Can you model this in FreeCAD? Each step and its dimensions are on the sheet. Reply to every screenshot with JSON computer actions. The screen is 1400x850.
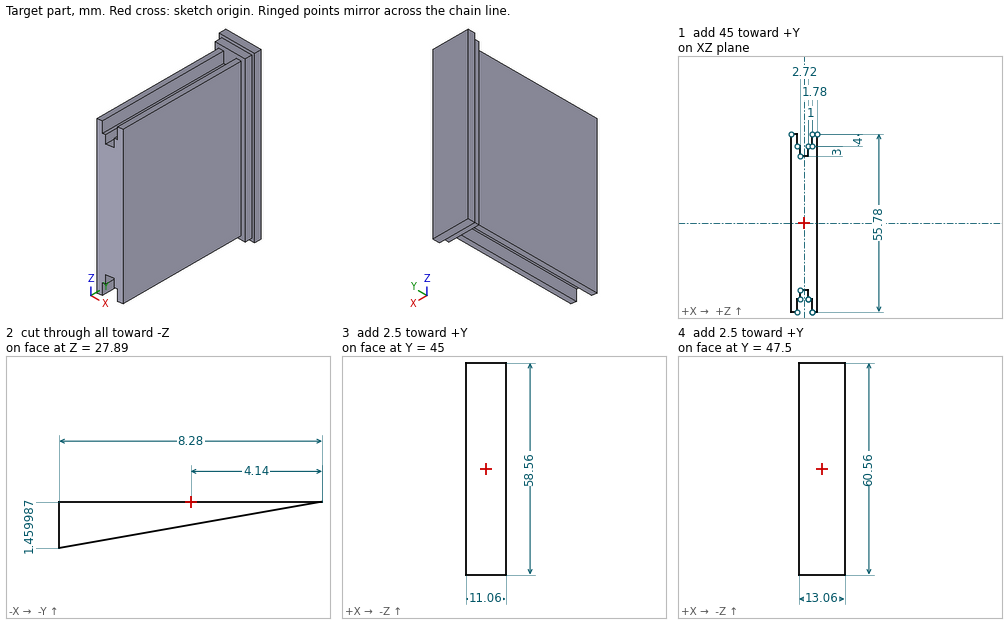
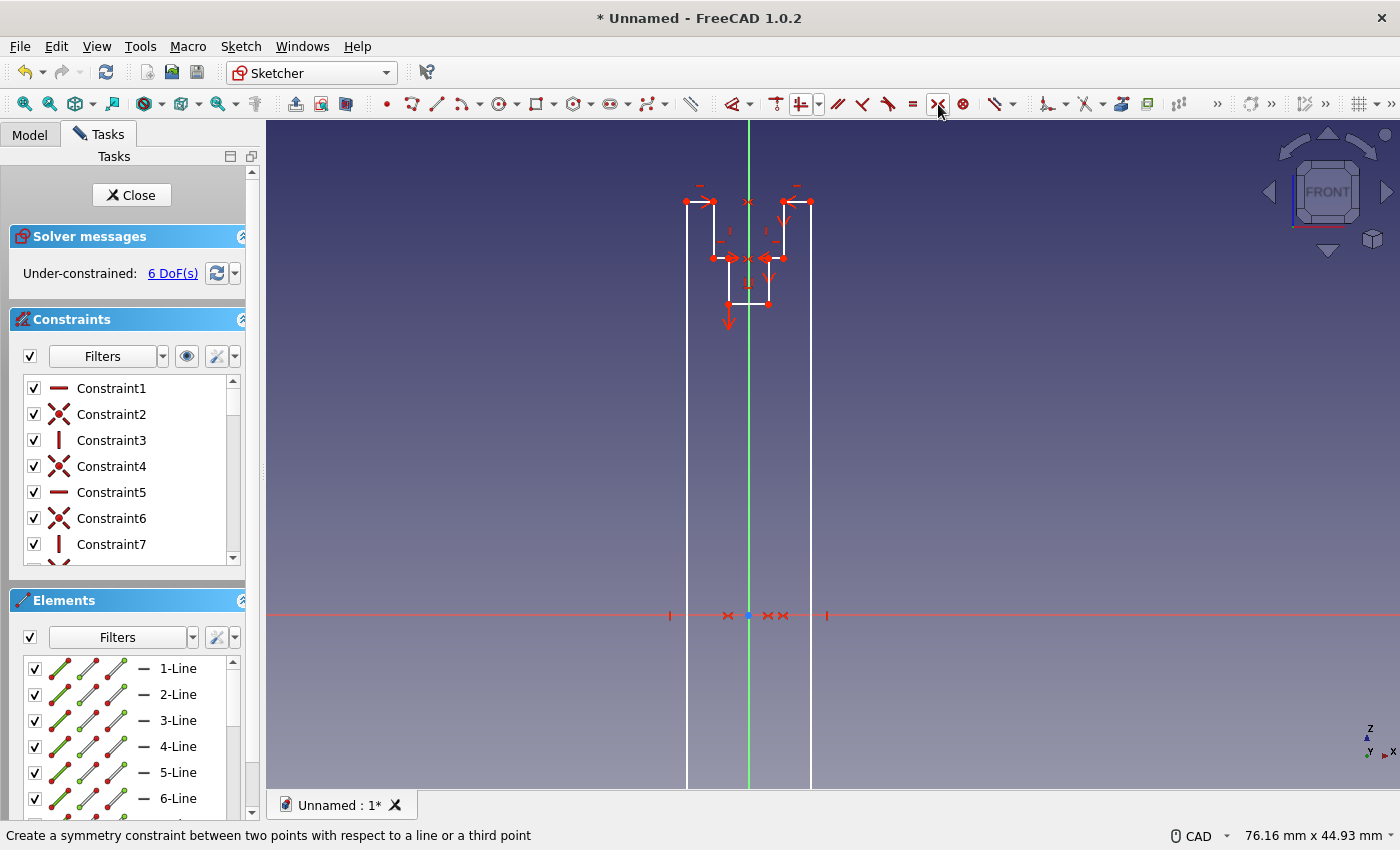
{"action": "left_click", "coordinate": [732, 104]}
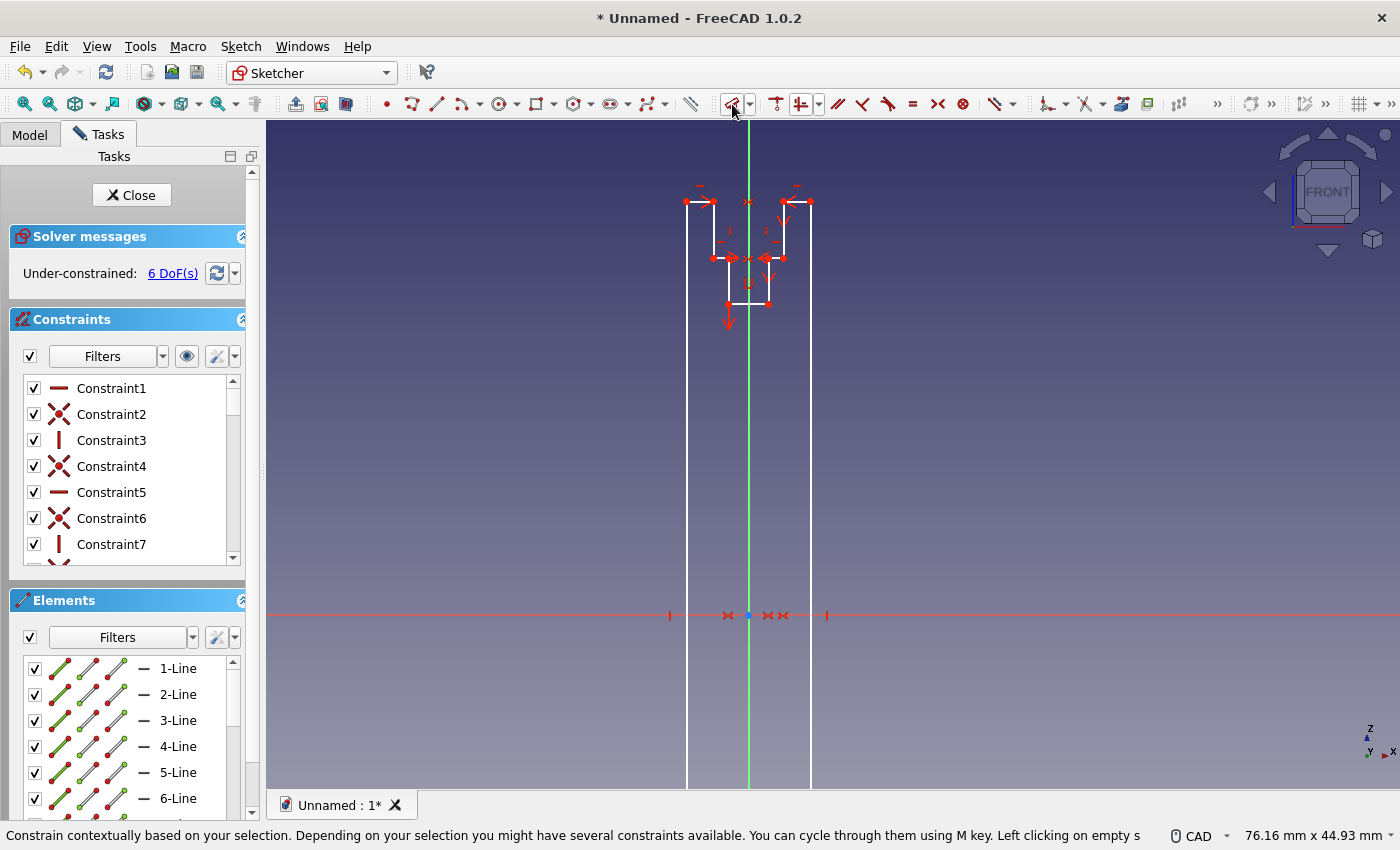
{"action": "left_click", "coordinate": [769, 290]}
{"action": "left_click", "coordinate": [827, 281]}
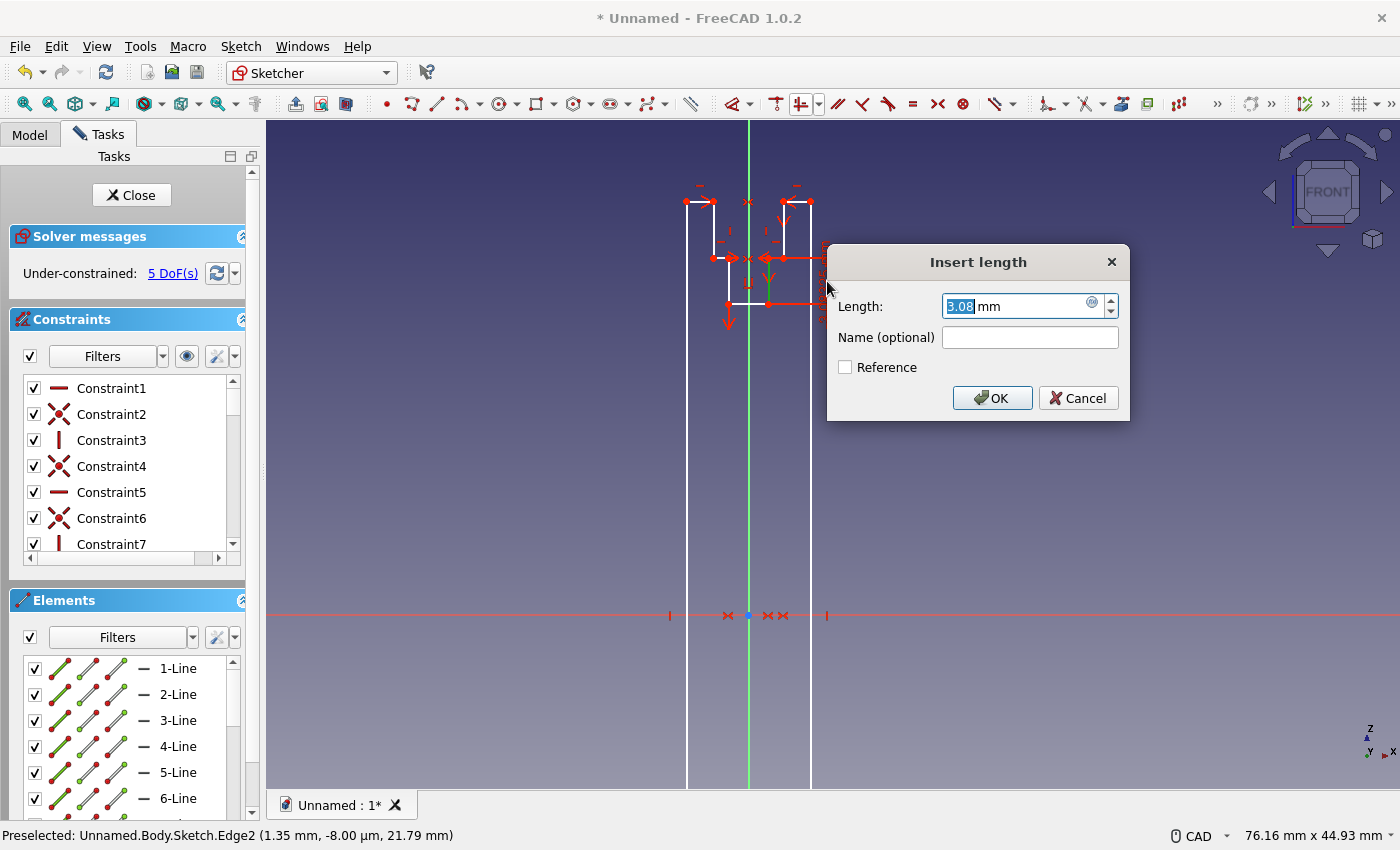
{"action": "type", "text": "3"}
{"action": "key", "text": "Return"}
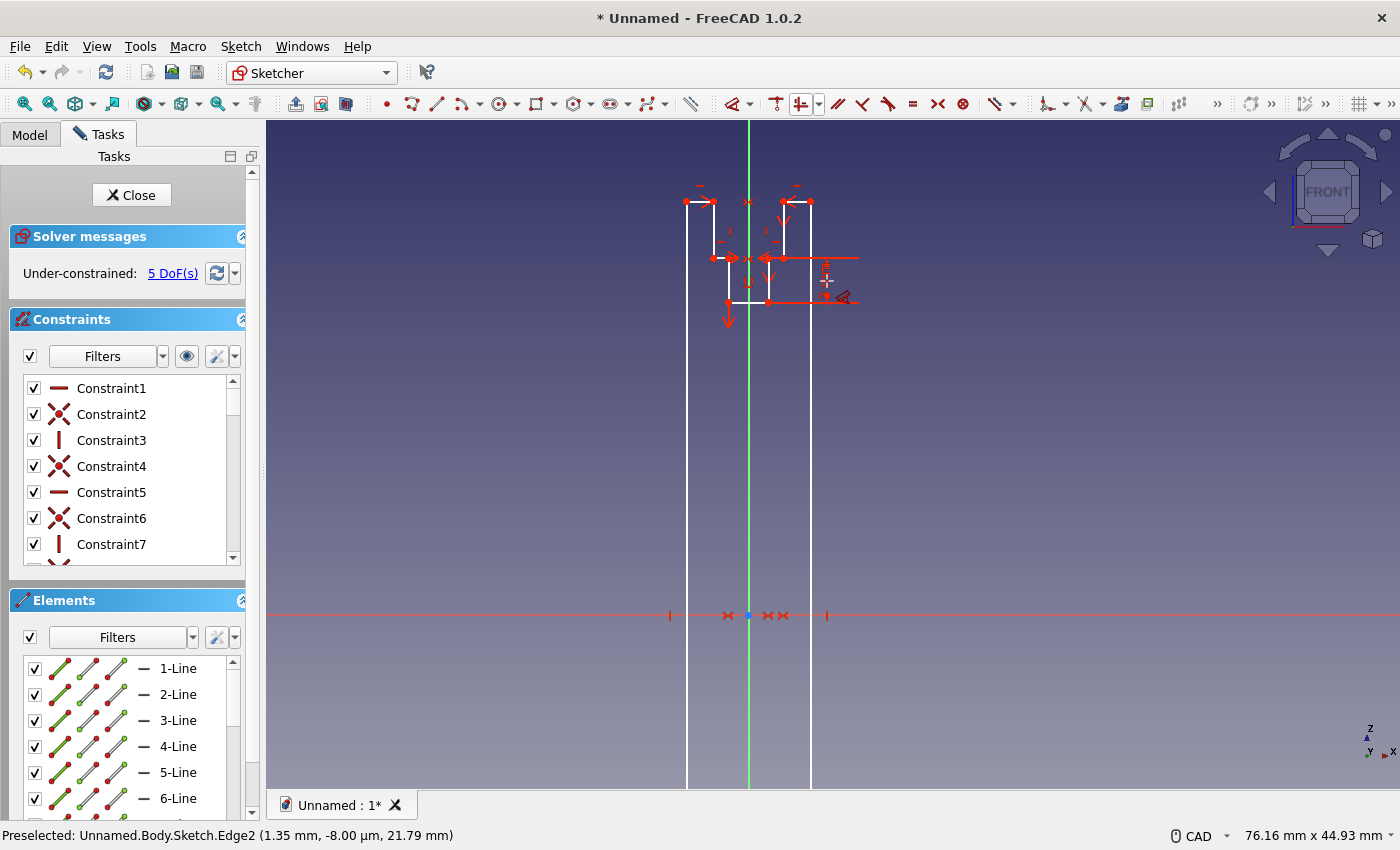
{"action": "scroll", "coordinate": [776, 258], "scroll_direction": "up", "scroll_amount": 5}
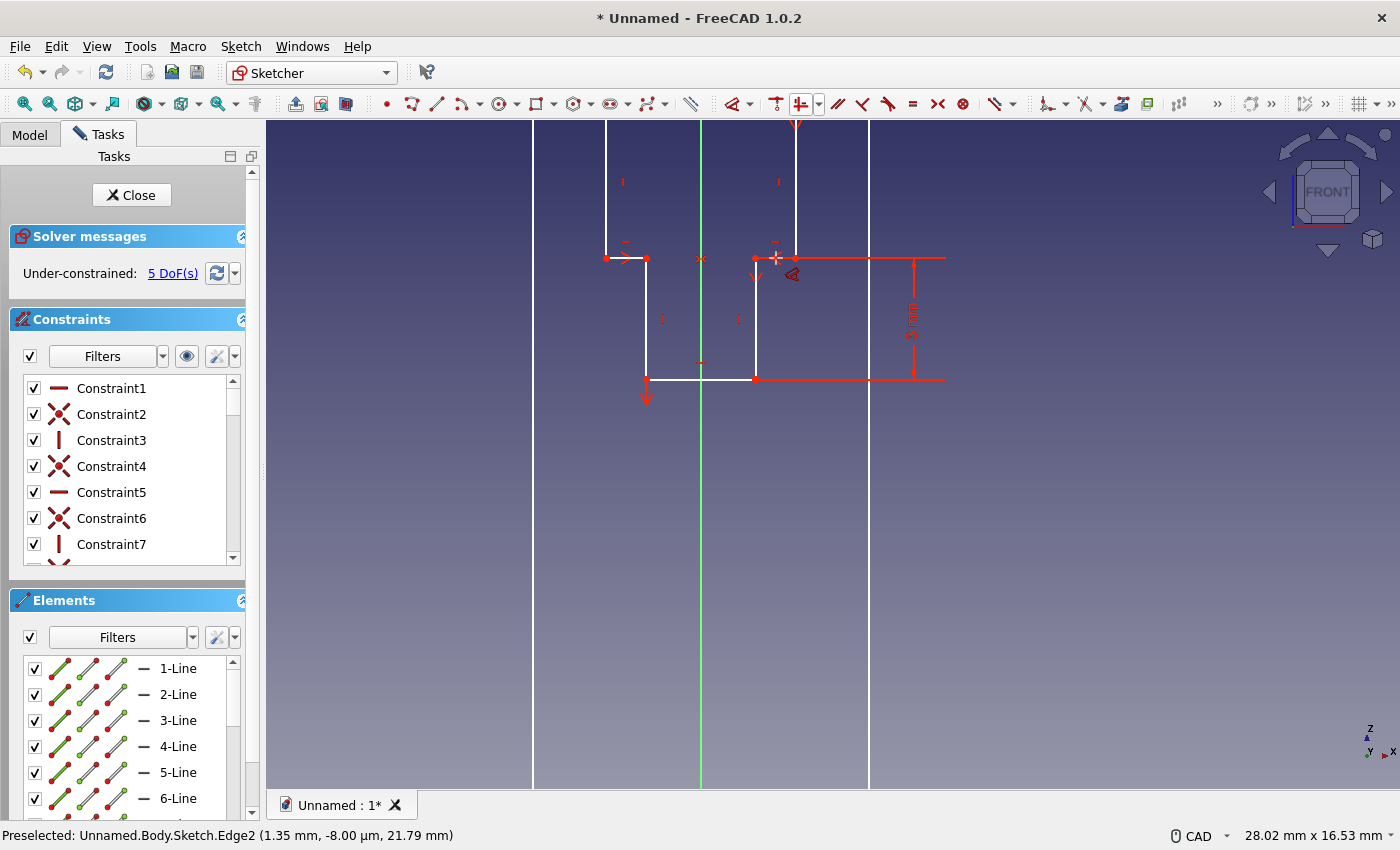
{"action": "left_click", "coordinate": [776, 258]}
{"action": "left_click", "coordinate": [776, 224]}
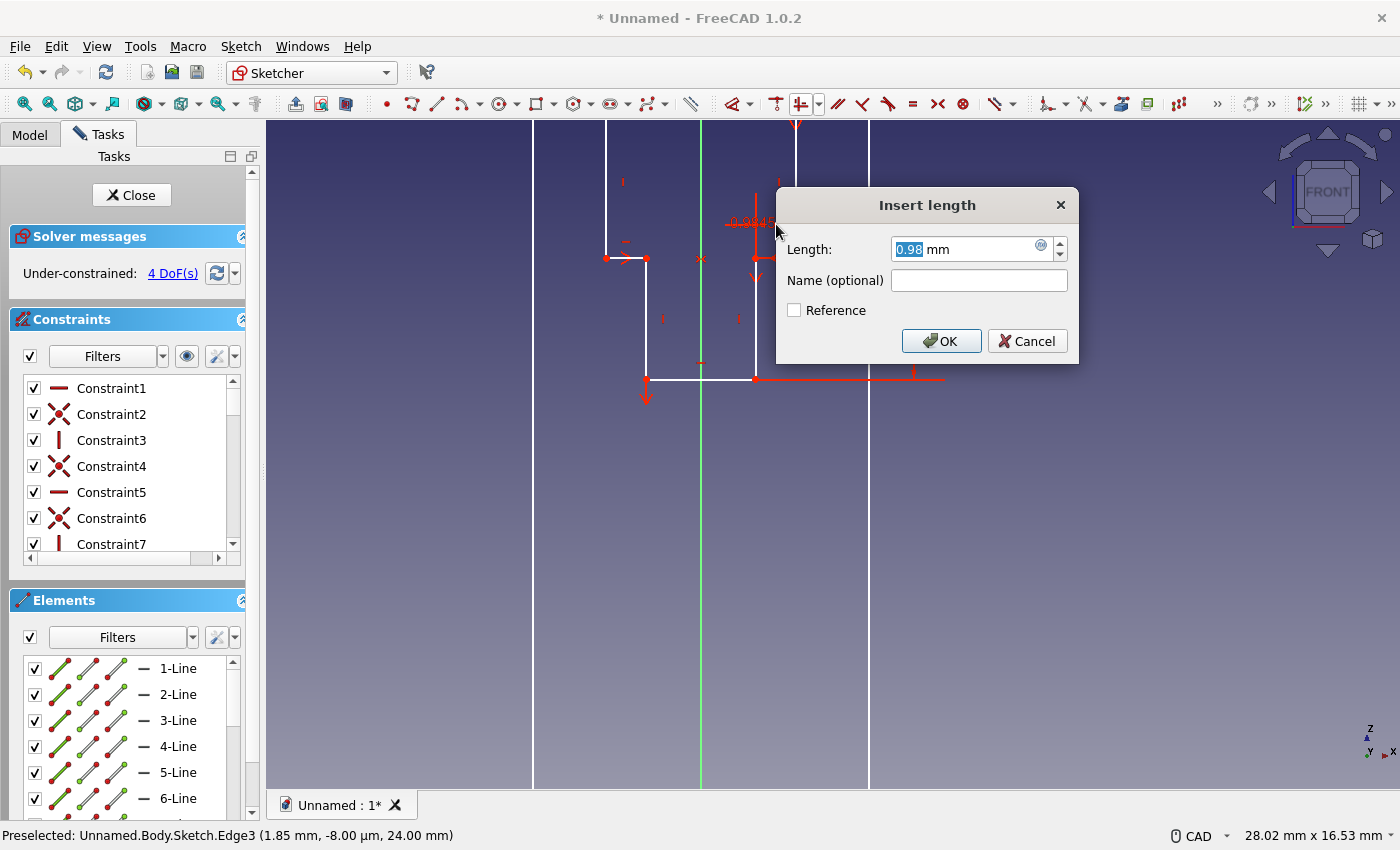
{"action": "type", "text": "1"}
{"action": "key", "text": "Return"}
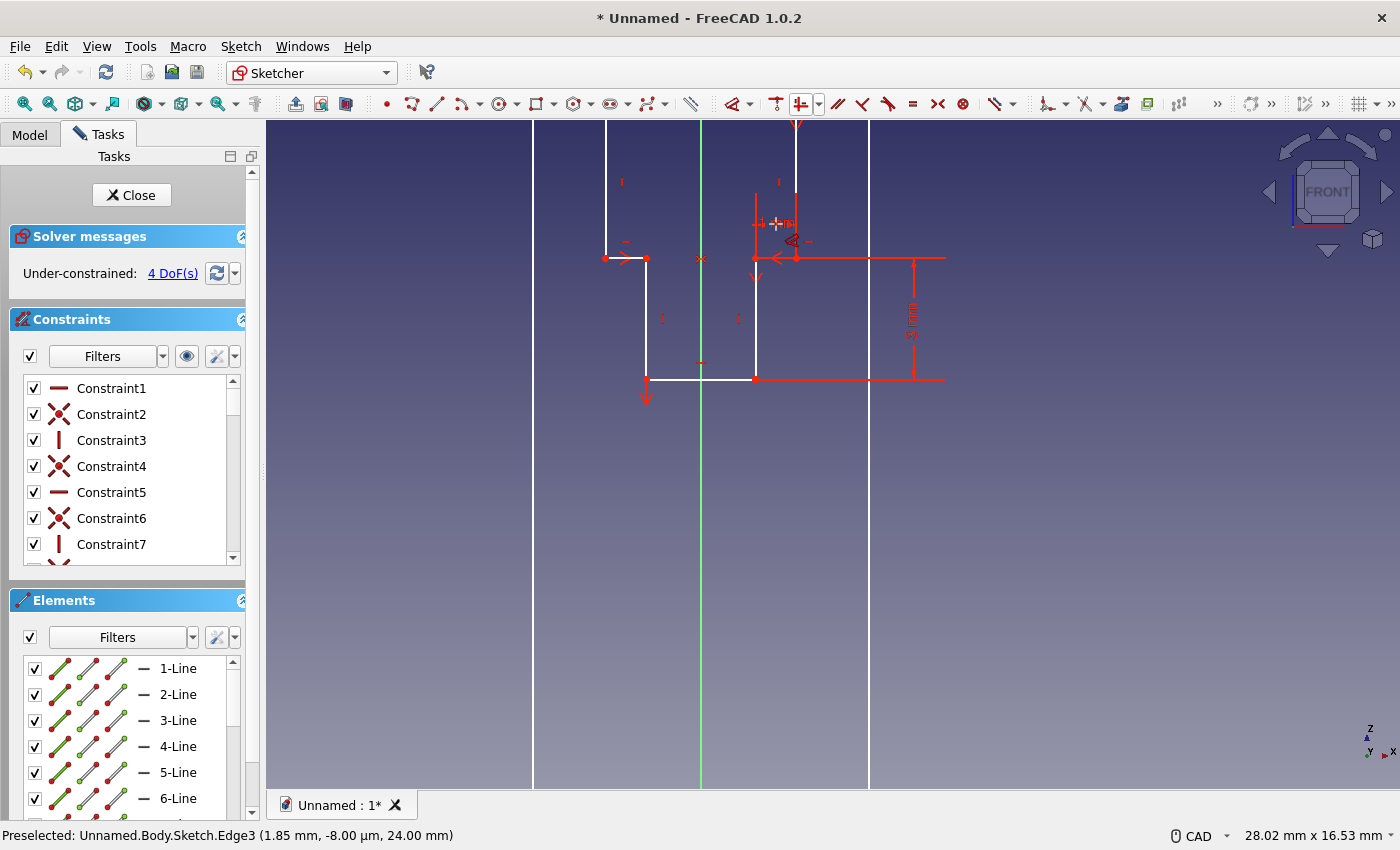
{"action": "scroll", "coordinate": [781, 258], "scroll_direction": "down", "scroll_amount": 8}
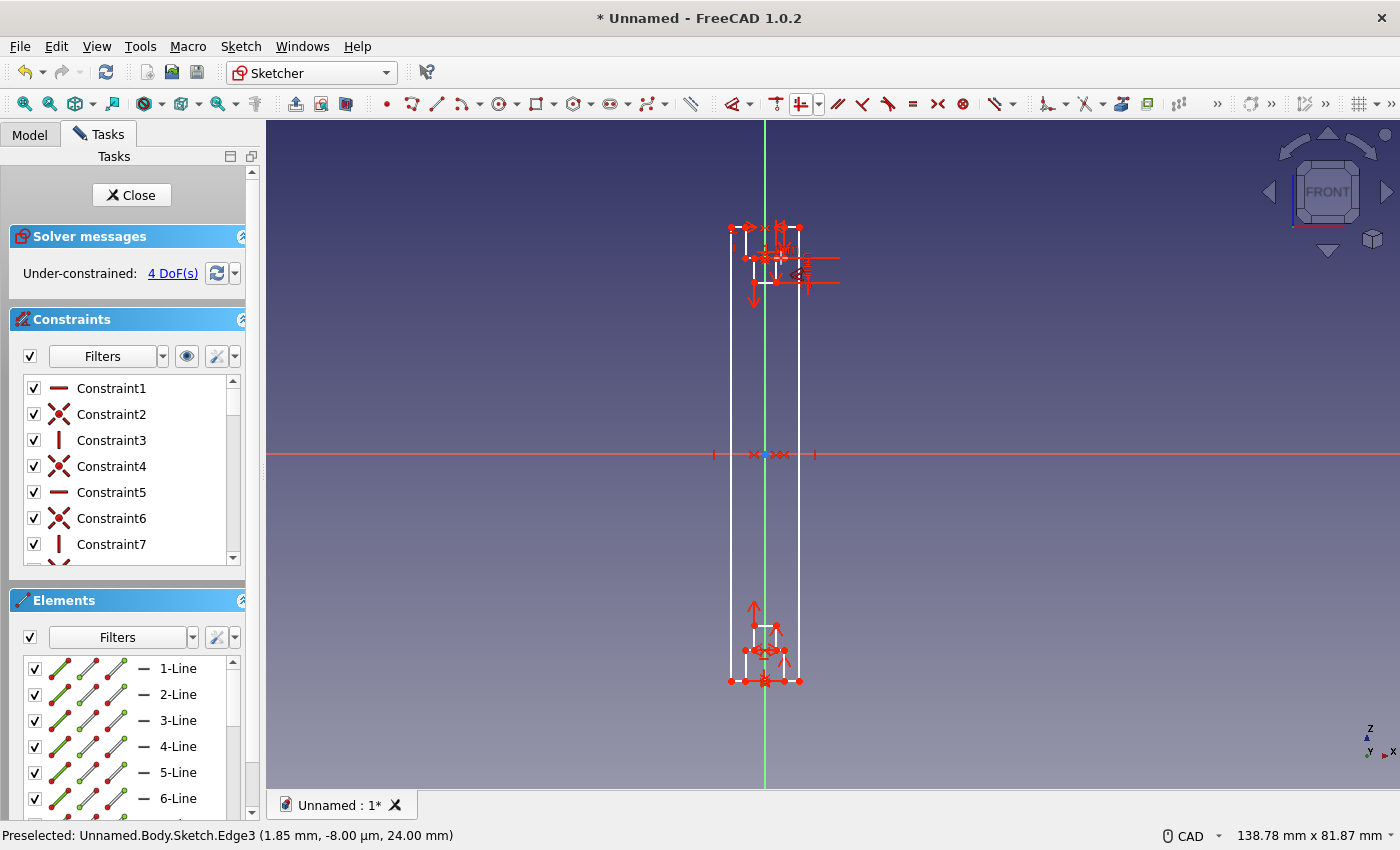
{"action": "scroll", "coordinate": [784, 249], "scroll_direction": "up", "scroll_amount": 2}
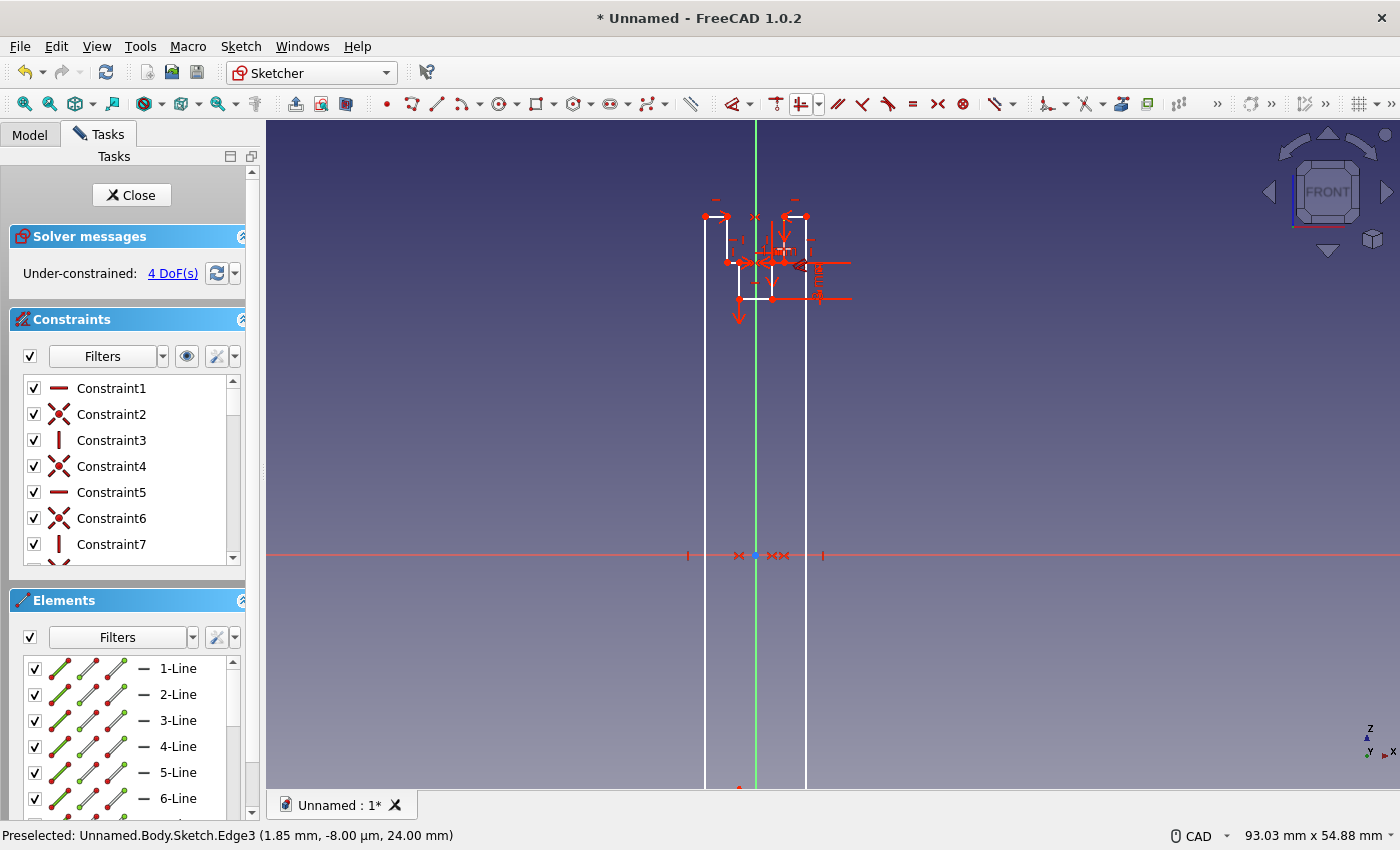
{"action": "left_click", "coordinate": [784, 249]}
{"action": "left_click", "coordinate": [842, 229]}